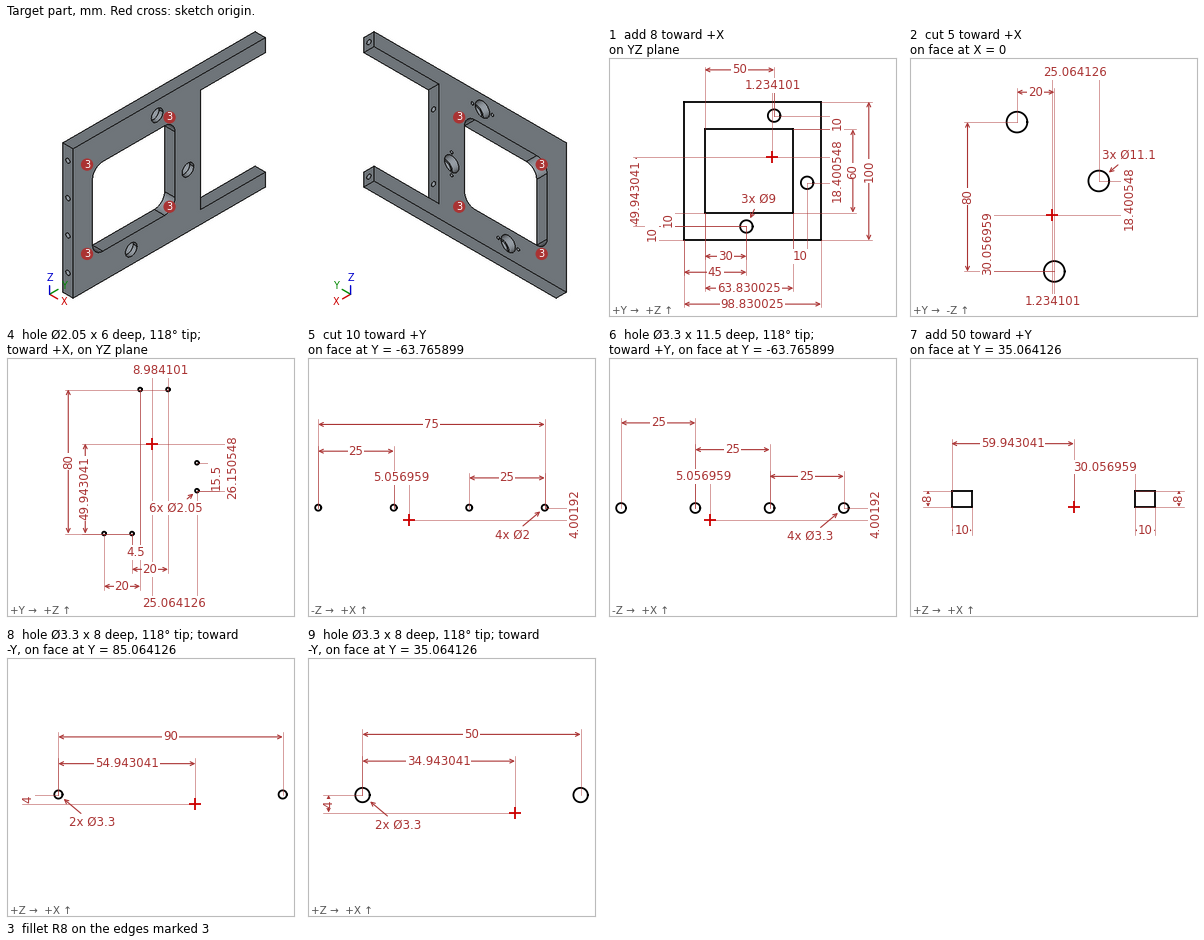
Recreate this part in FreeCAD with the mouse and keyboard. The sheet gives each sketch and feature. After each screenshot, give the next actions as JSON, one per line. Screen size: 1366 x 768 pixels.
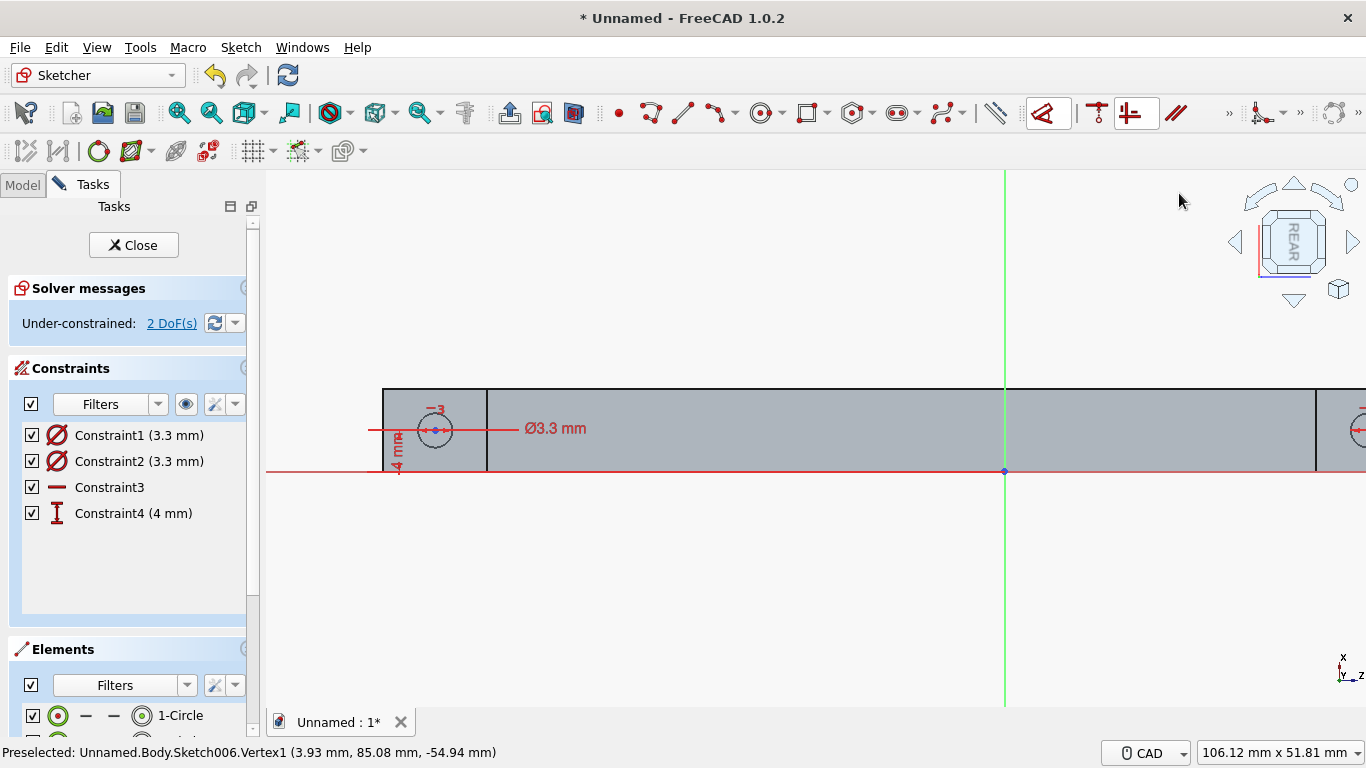
{"action": "left_click", "coordinate": [435, 430]}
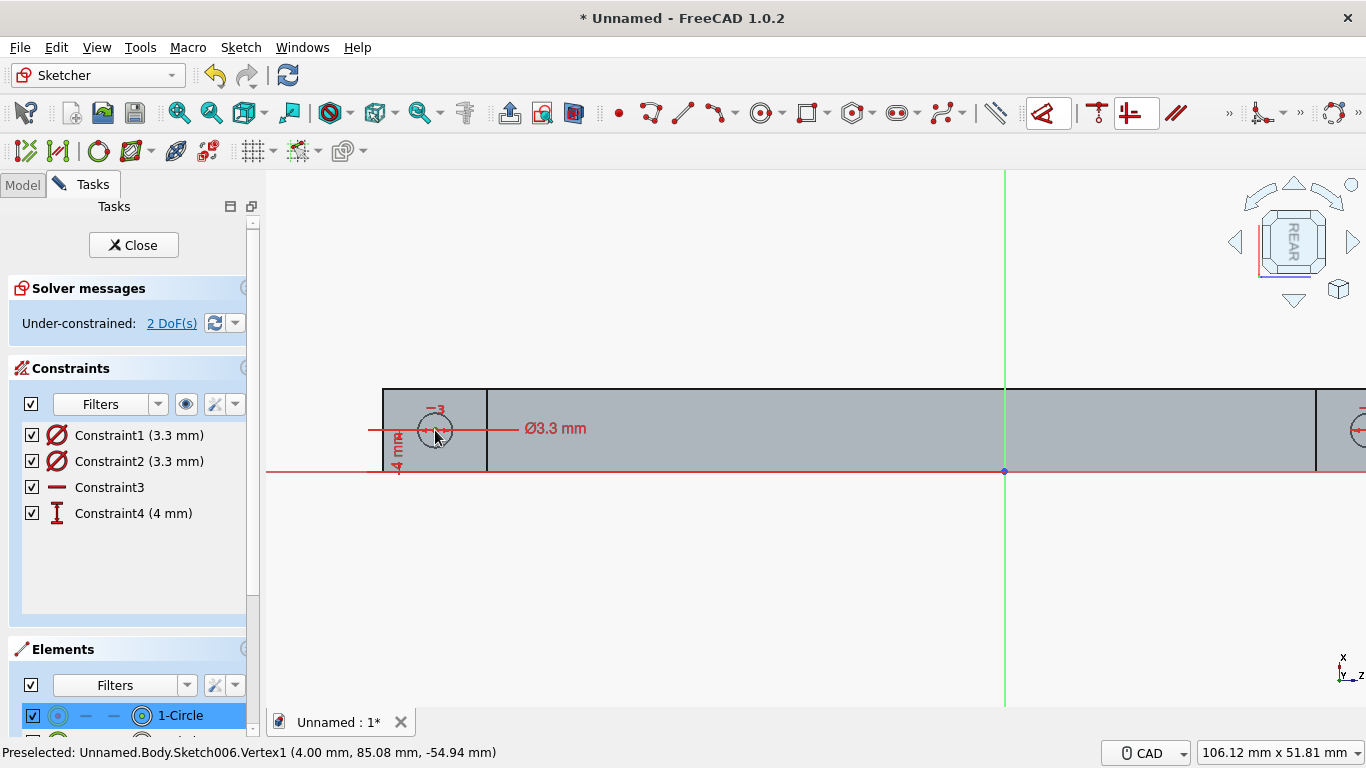
{"action": "scroll", "coordinate": [434, 430], "scroll_direction": "down", "scroll_amount": 2}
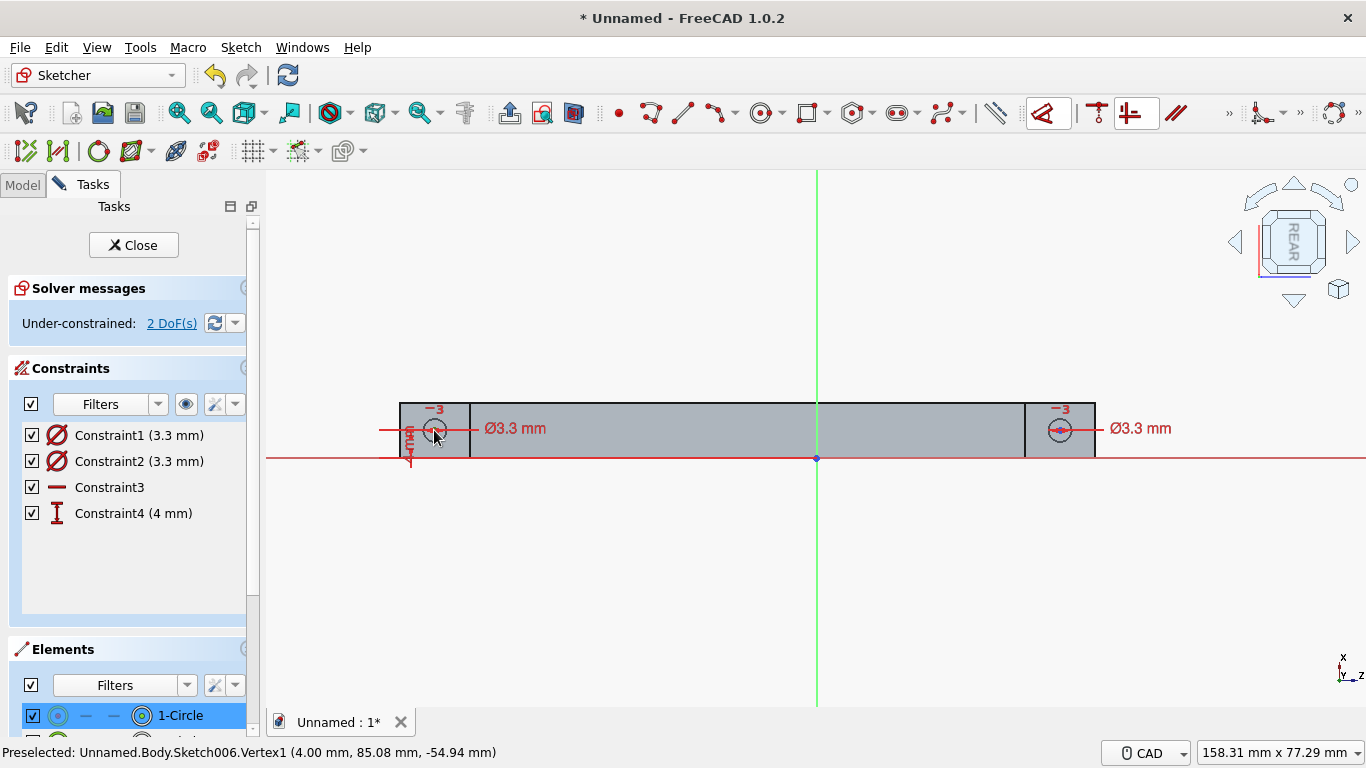
{"action": "left_click", "coordinate": [1060, 430]}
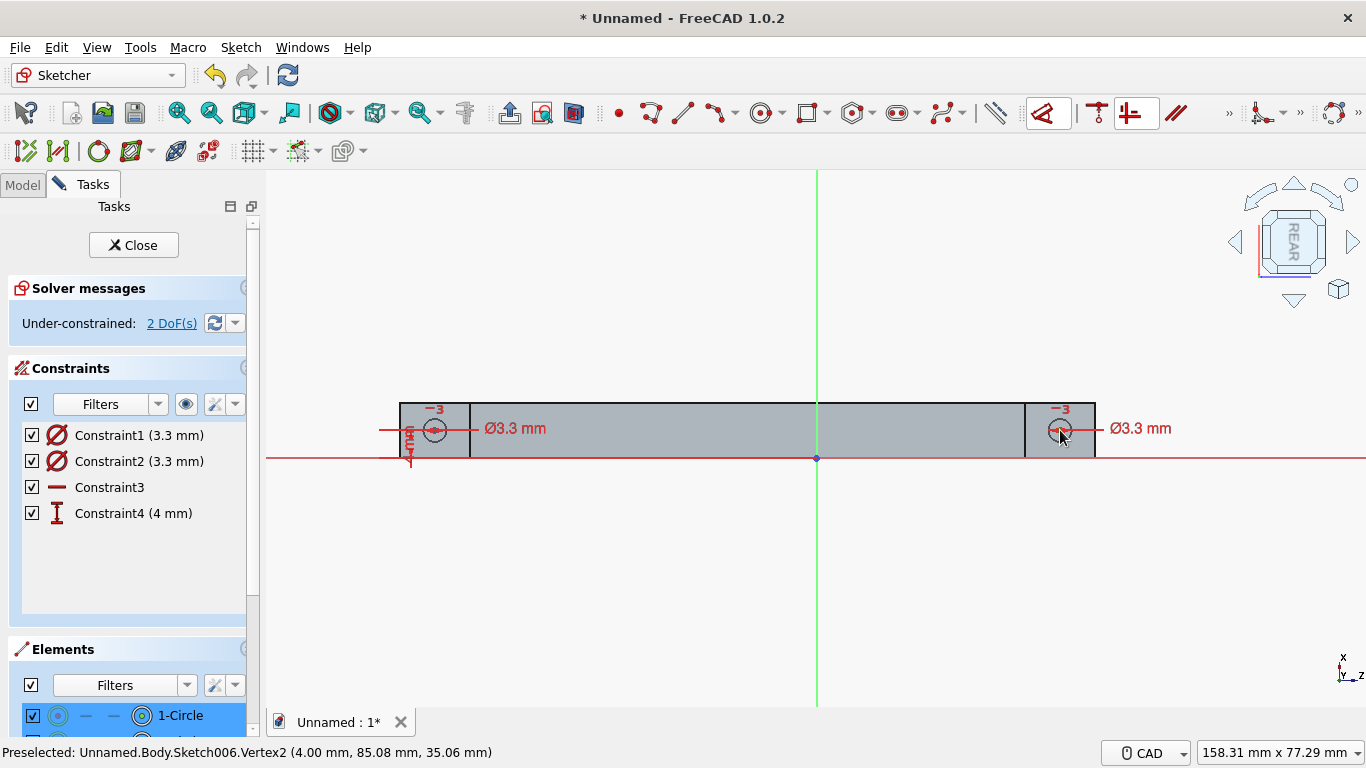
{"action": "key", "text": "l"}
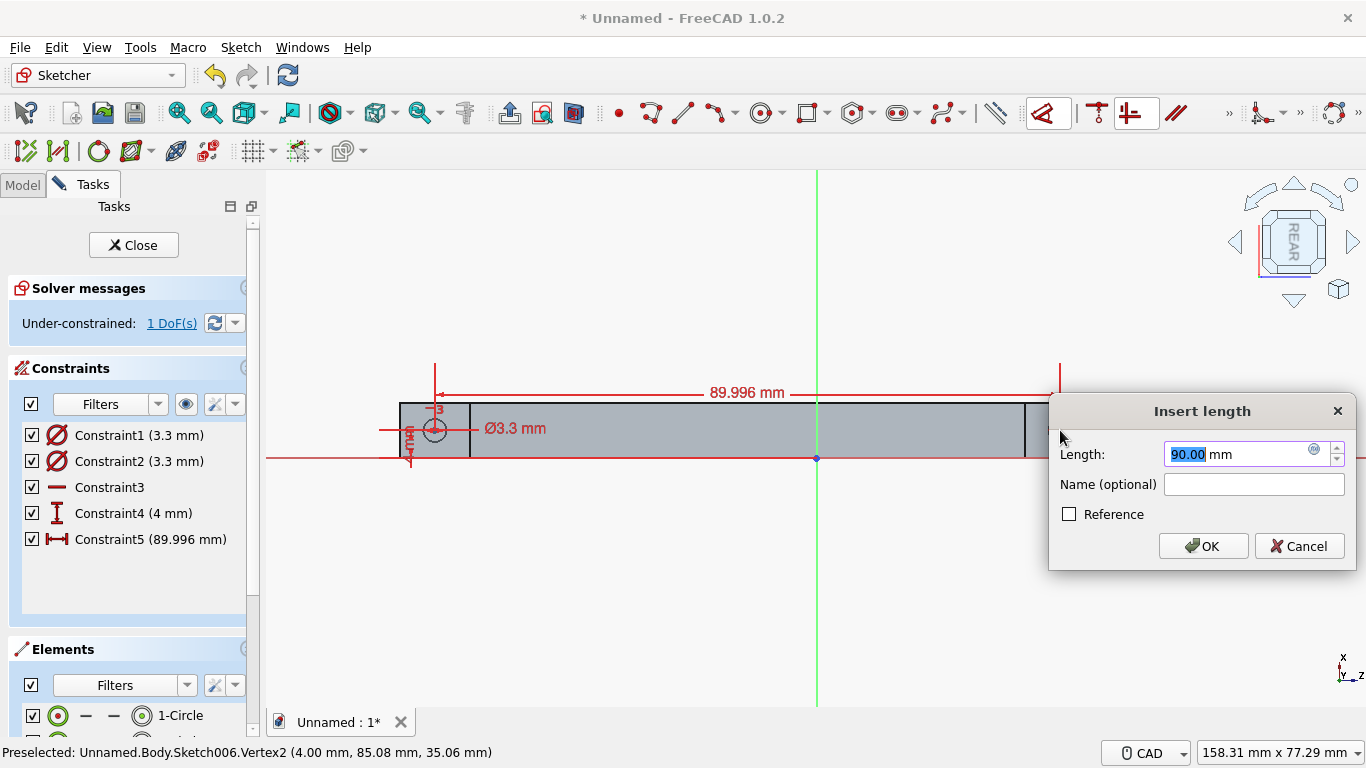
{"action": "type", "text": "90"}
{"action": "key", "text": "Return"}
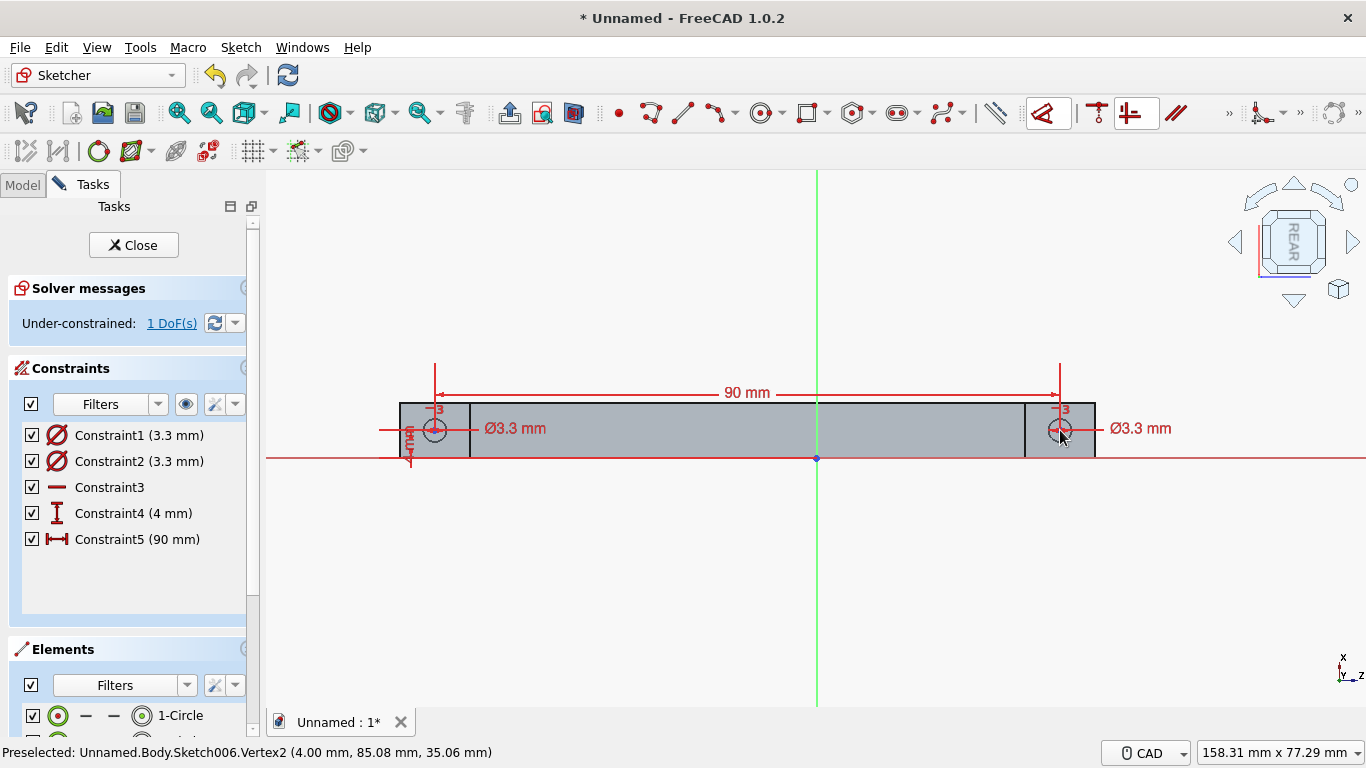
{"action": "left_click", "coordinate": [435, 430]}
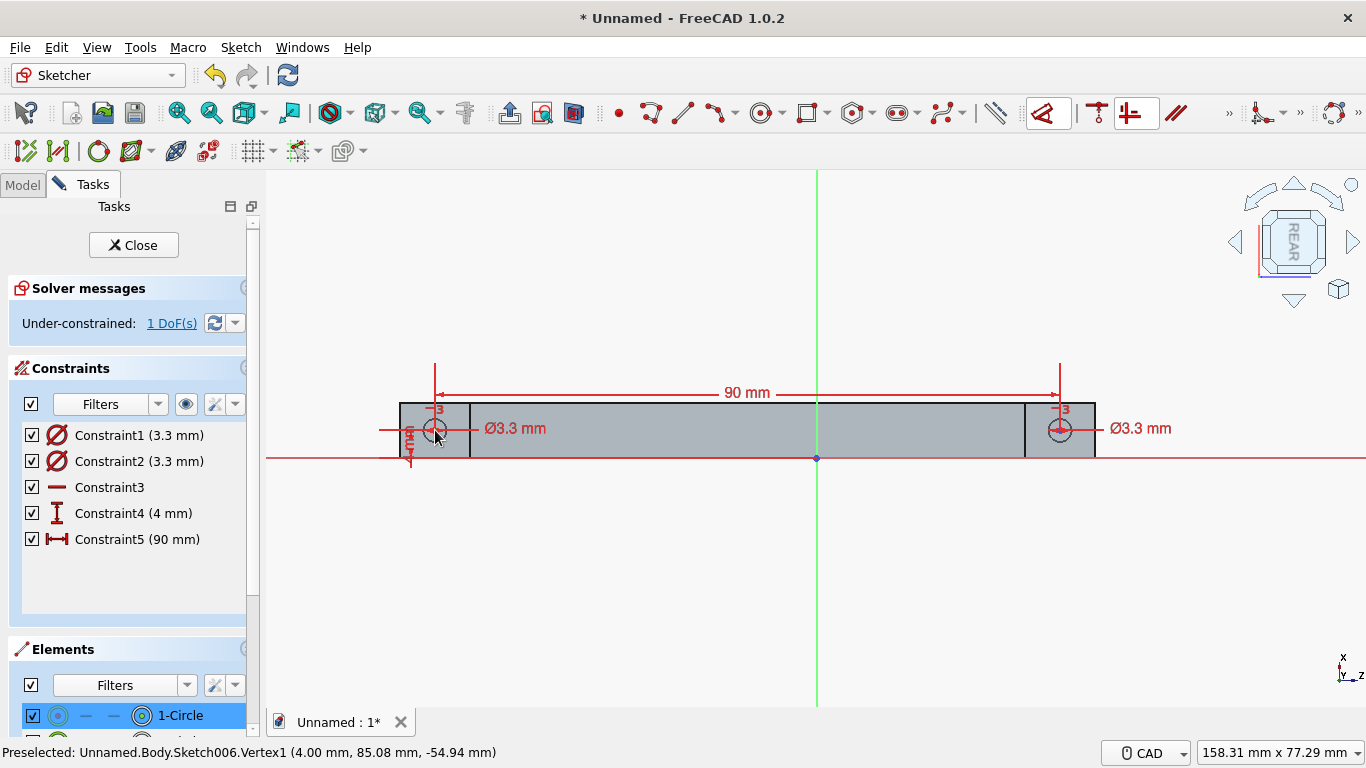
{"action": "key", "text": "l"}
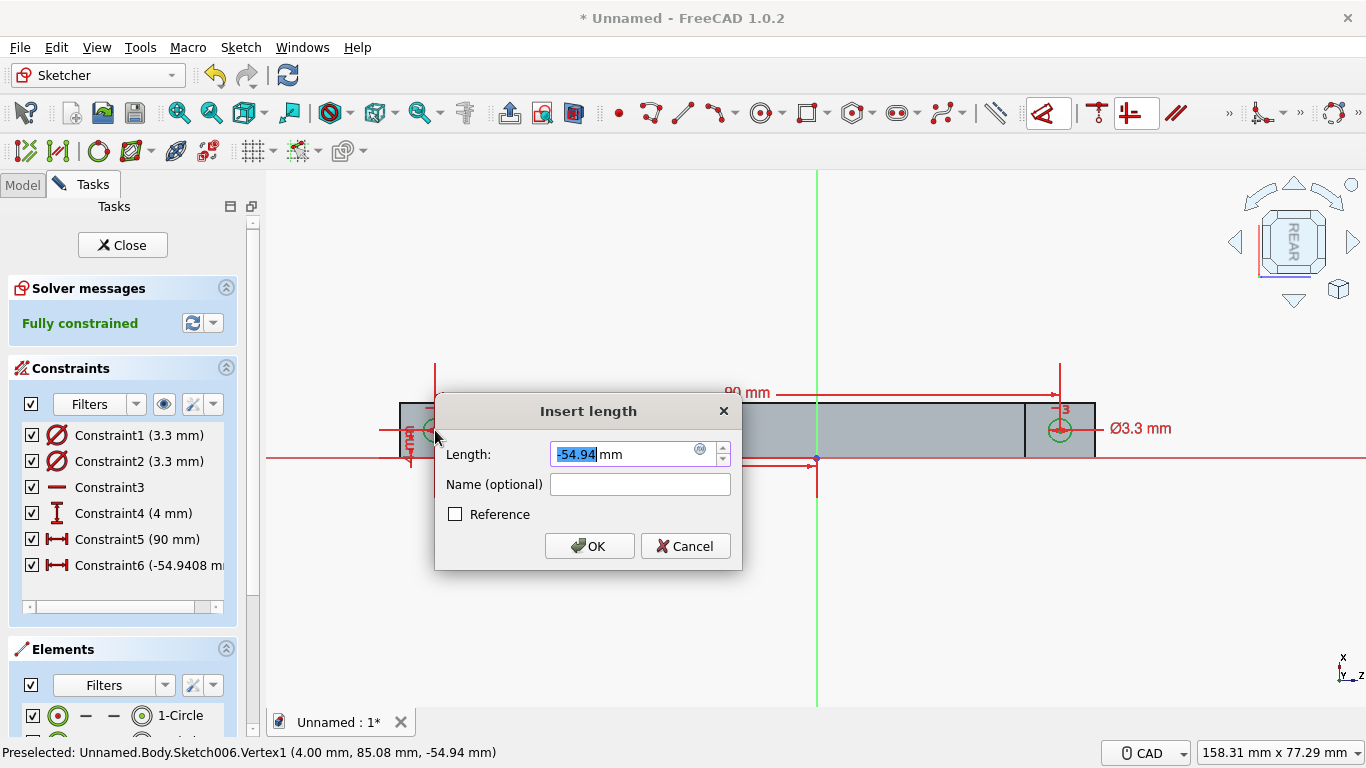
{"action": "type", "text": "-54.943041"}
{"action": "key", "text": "Return"}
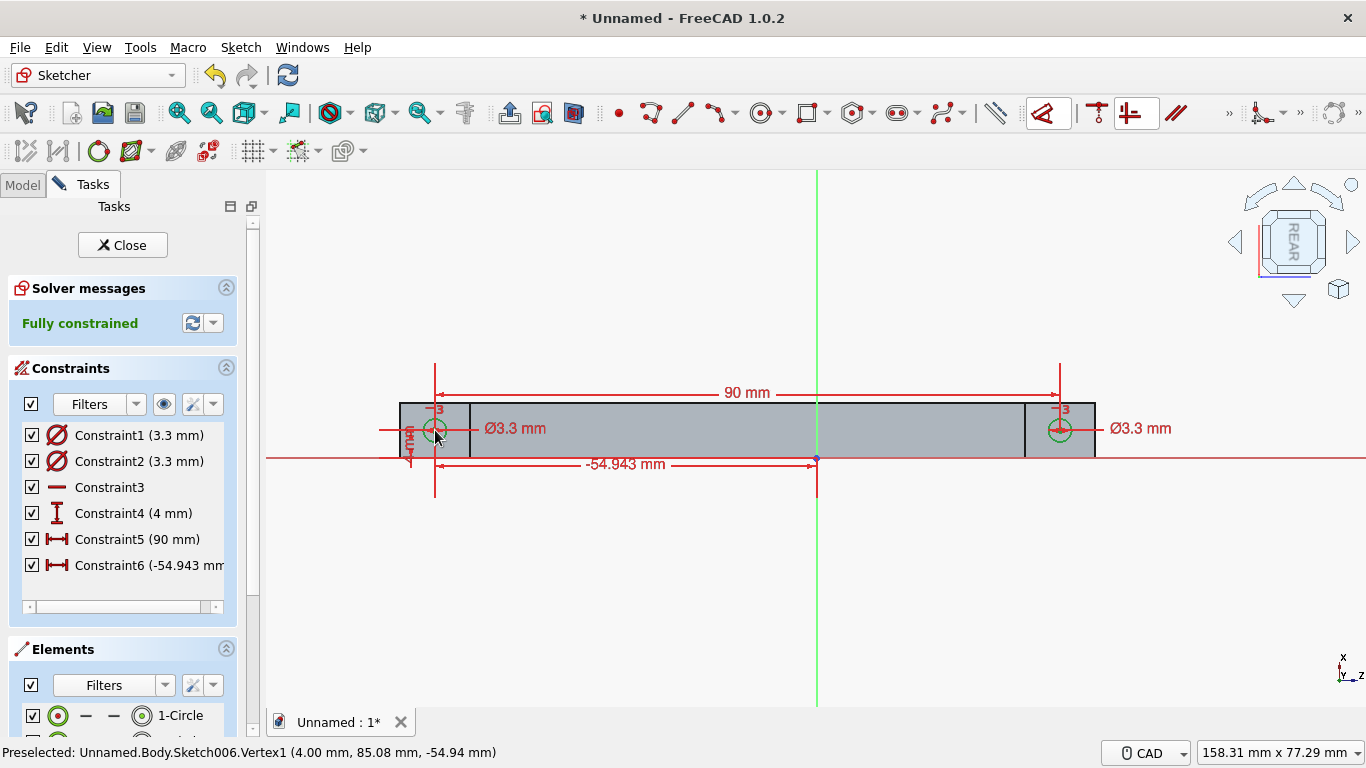
{"action": "left_click", "coordinate": [123, 245]}